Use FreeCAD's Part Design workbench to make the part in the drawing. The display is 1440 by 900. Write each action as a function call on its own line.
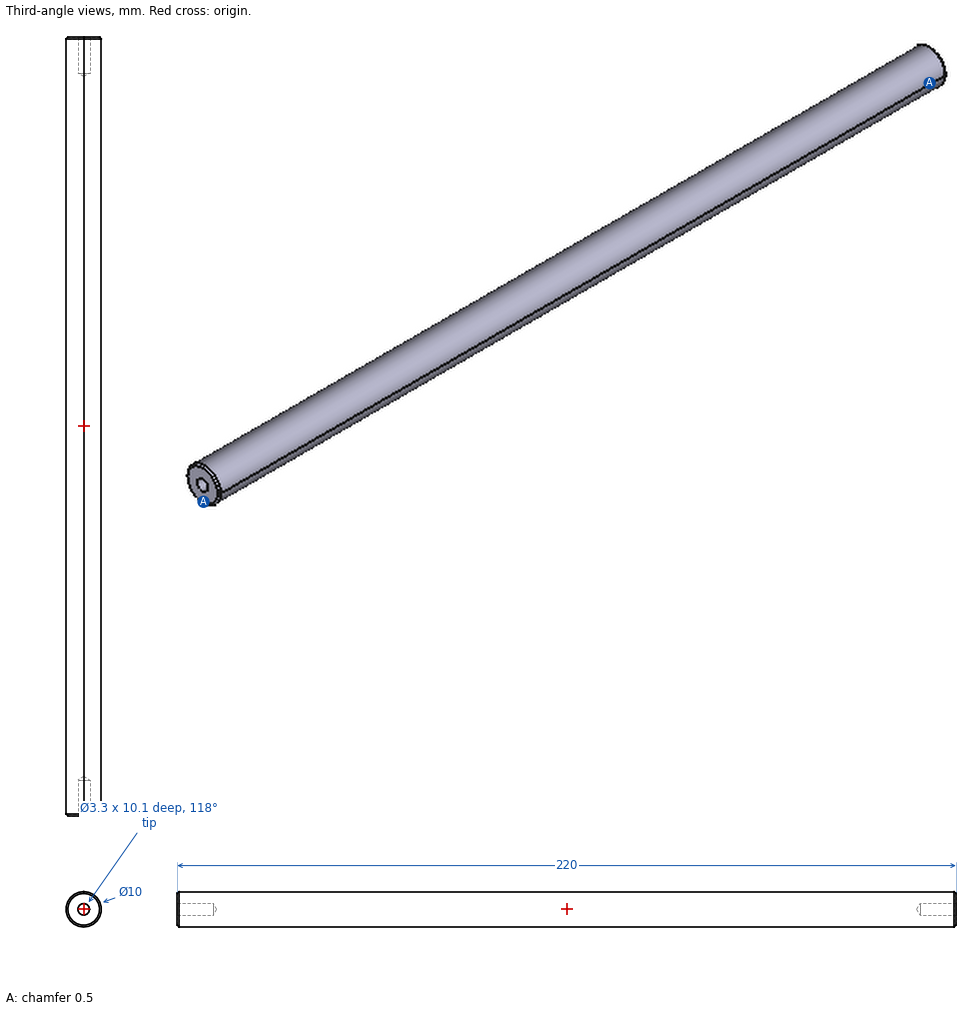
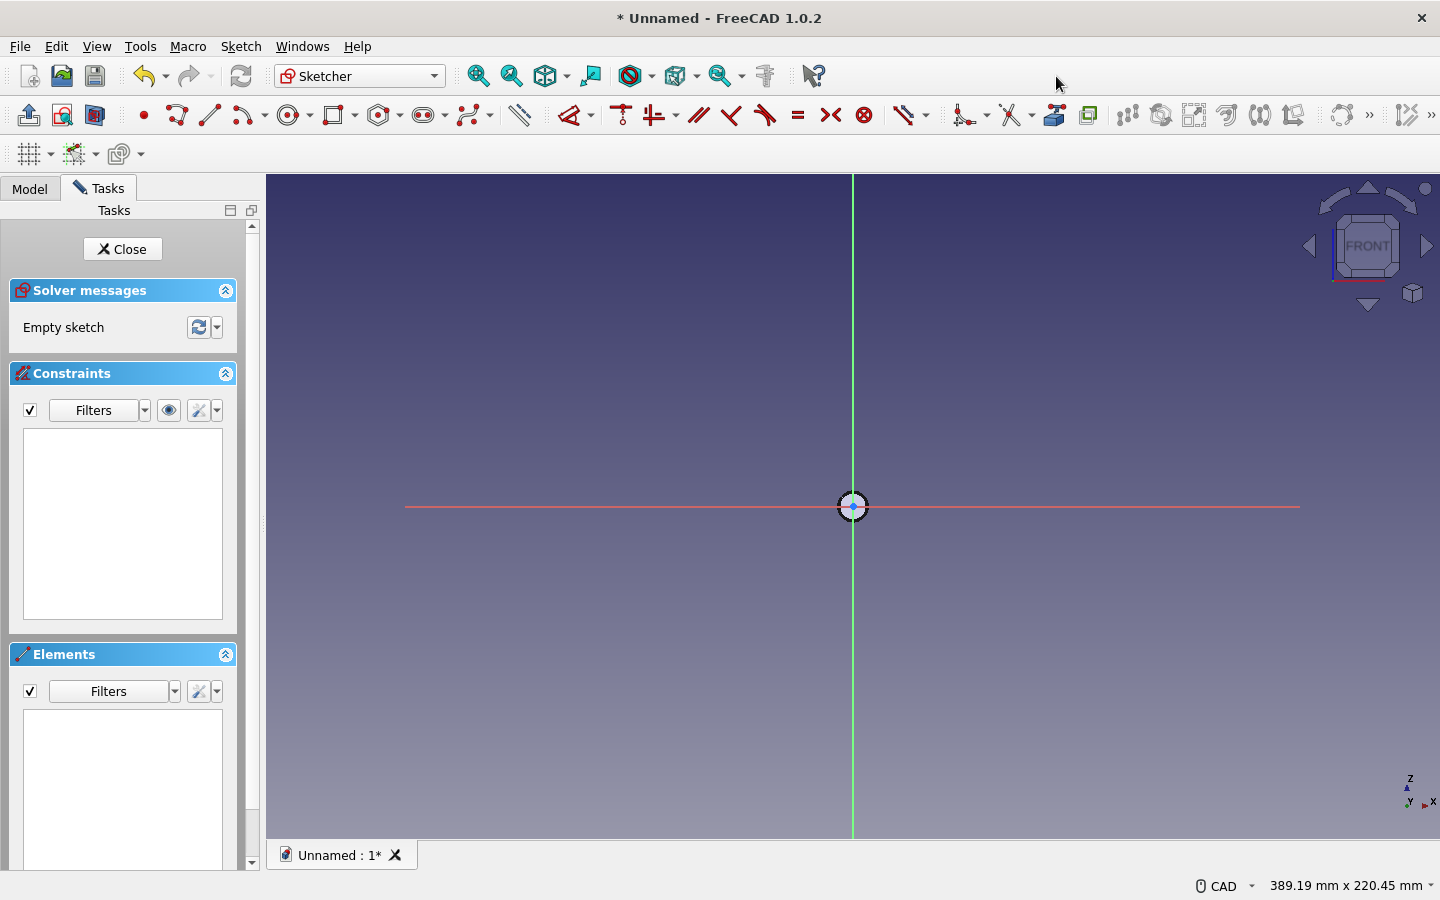
scroll(857, 506, up, 15)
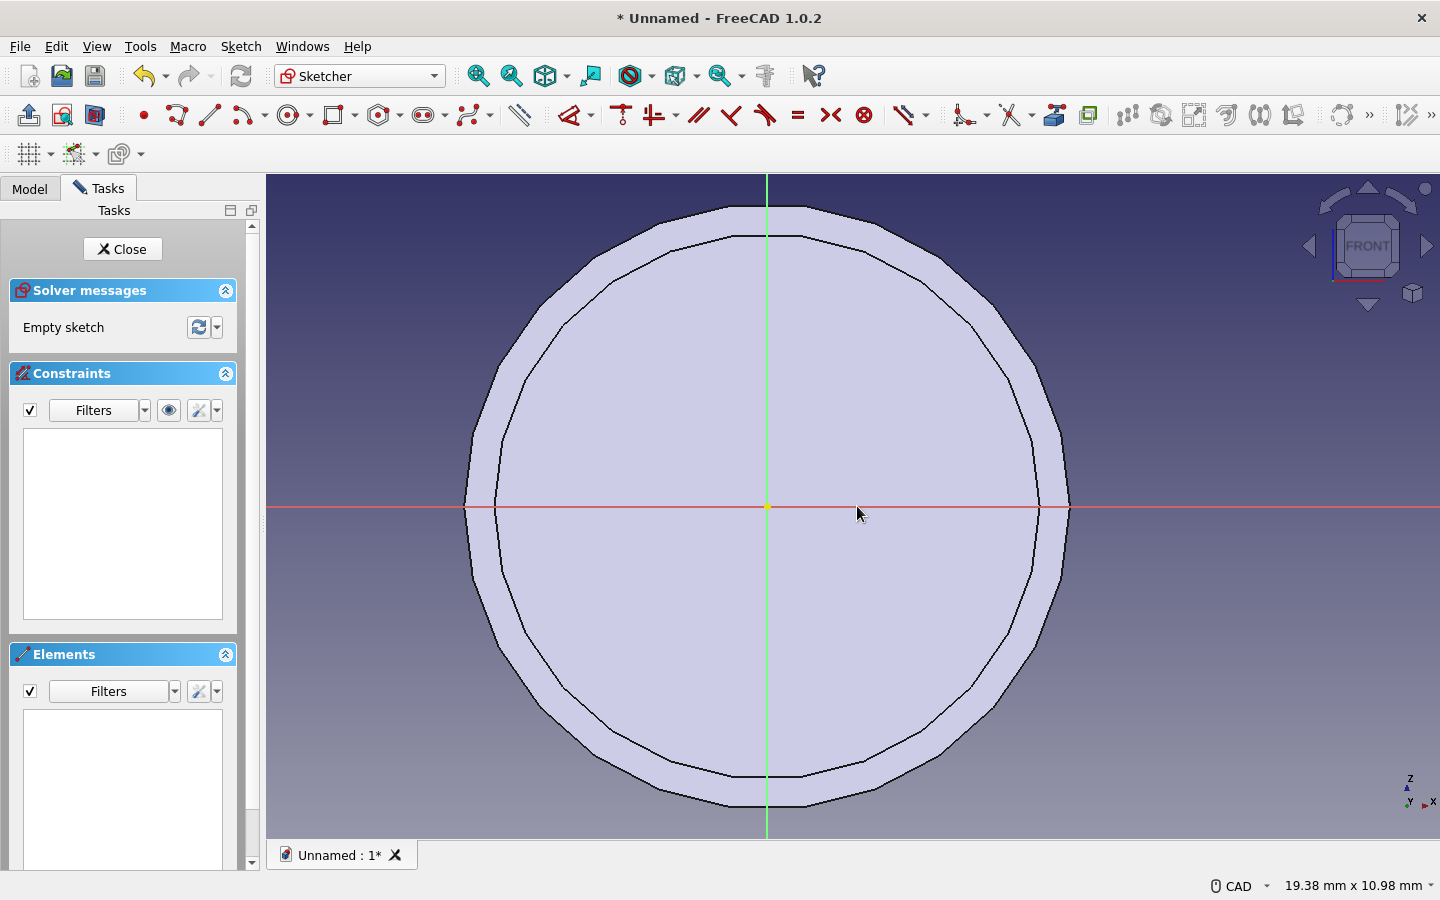
scroll(753, 506, up, 4)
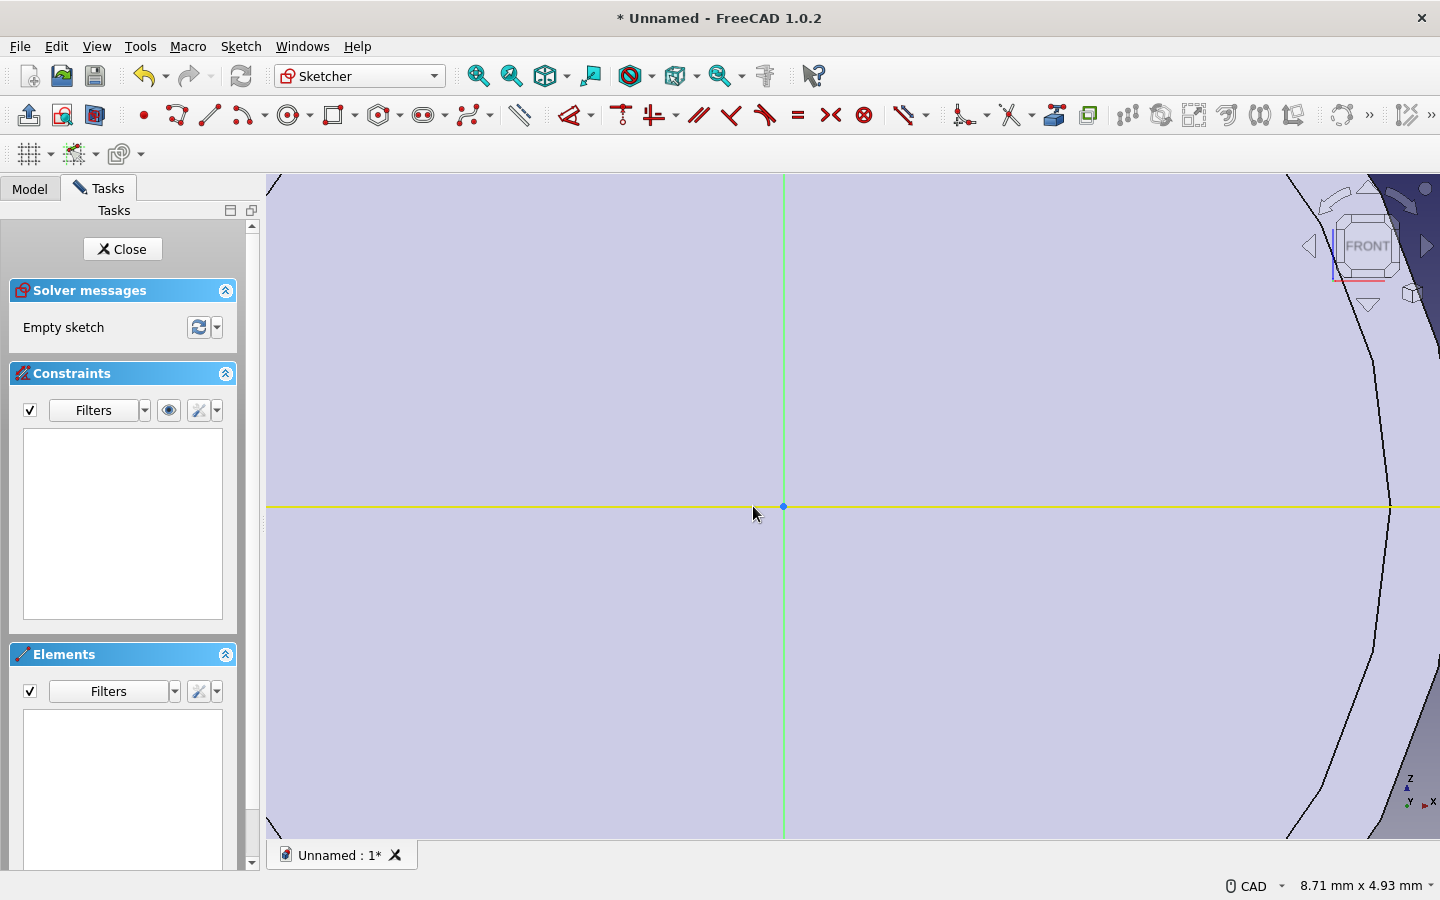
key(g)
key(c)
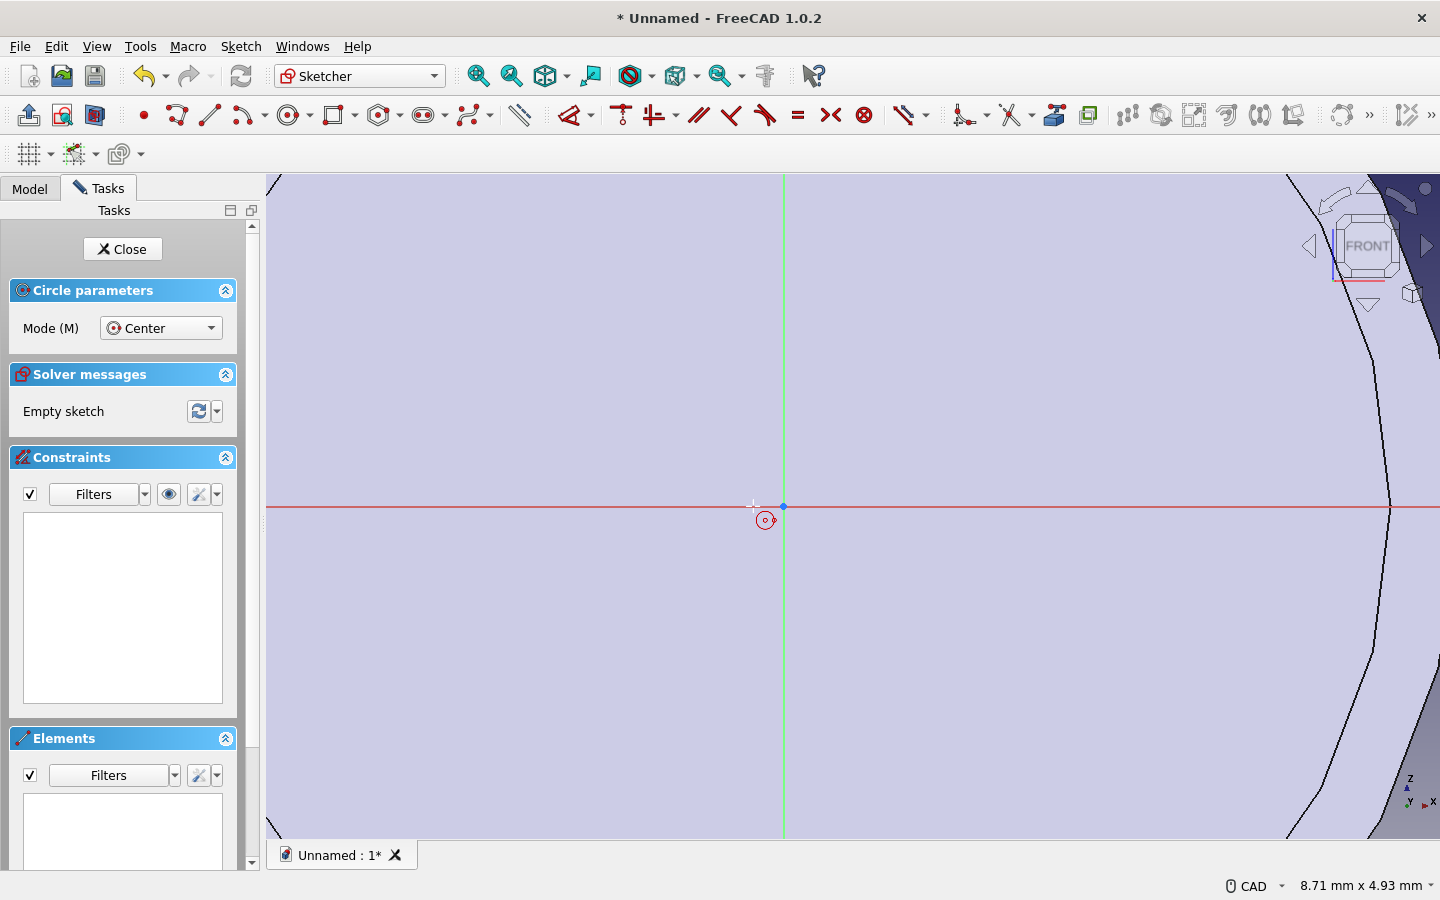
click(784, 506)
move(941, 349)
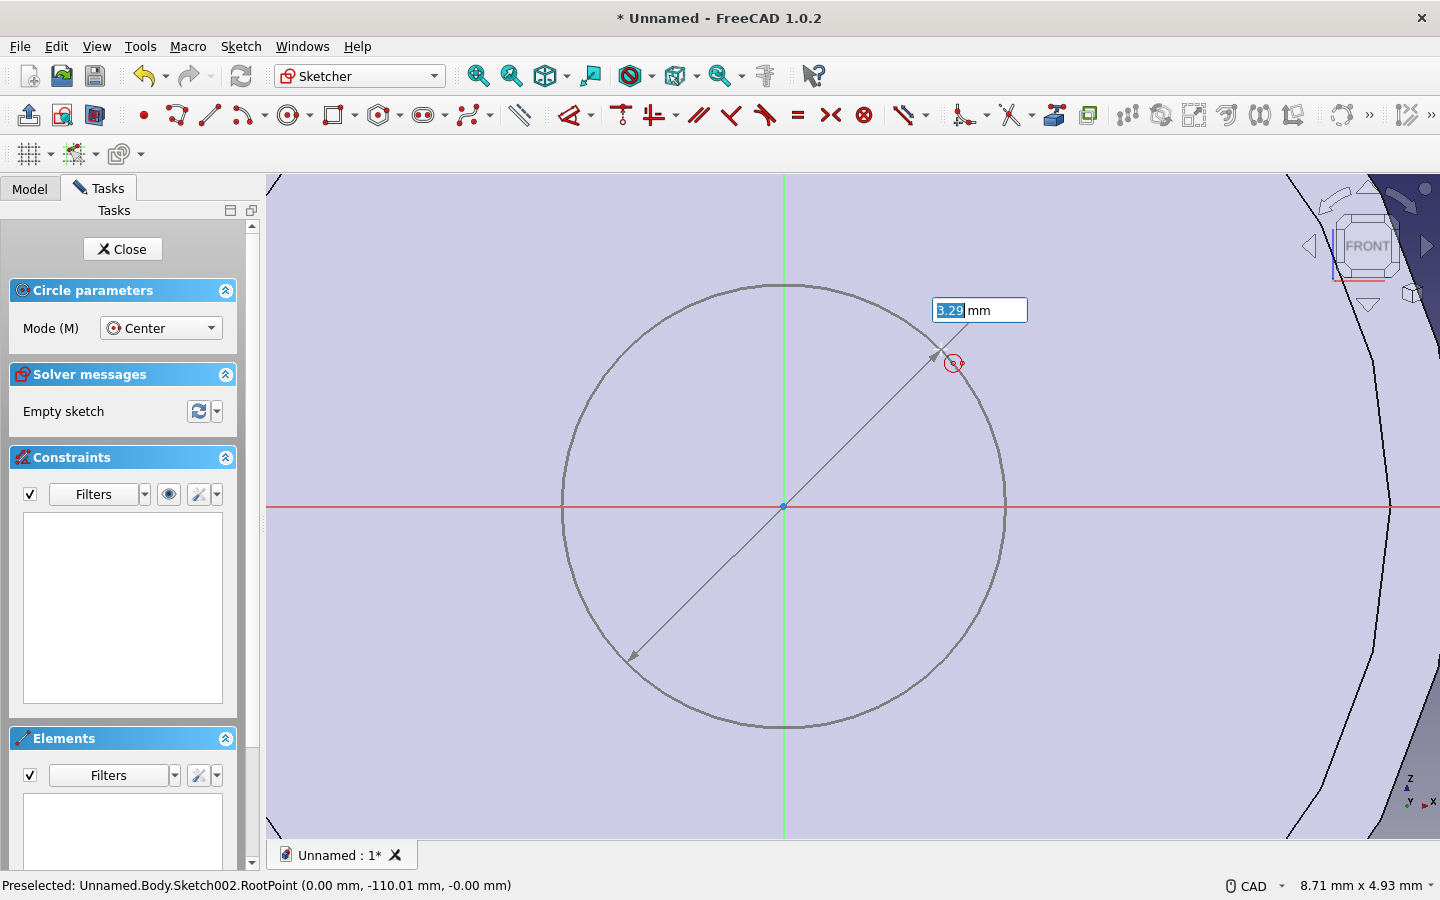
text(3.3)
key(Return)
key(Escape)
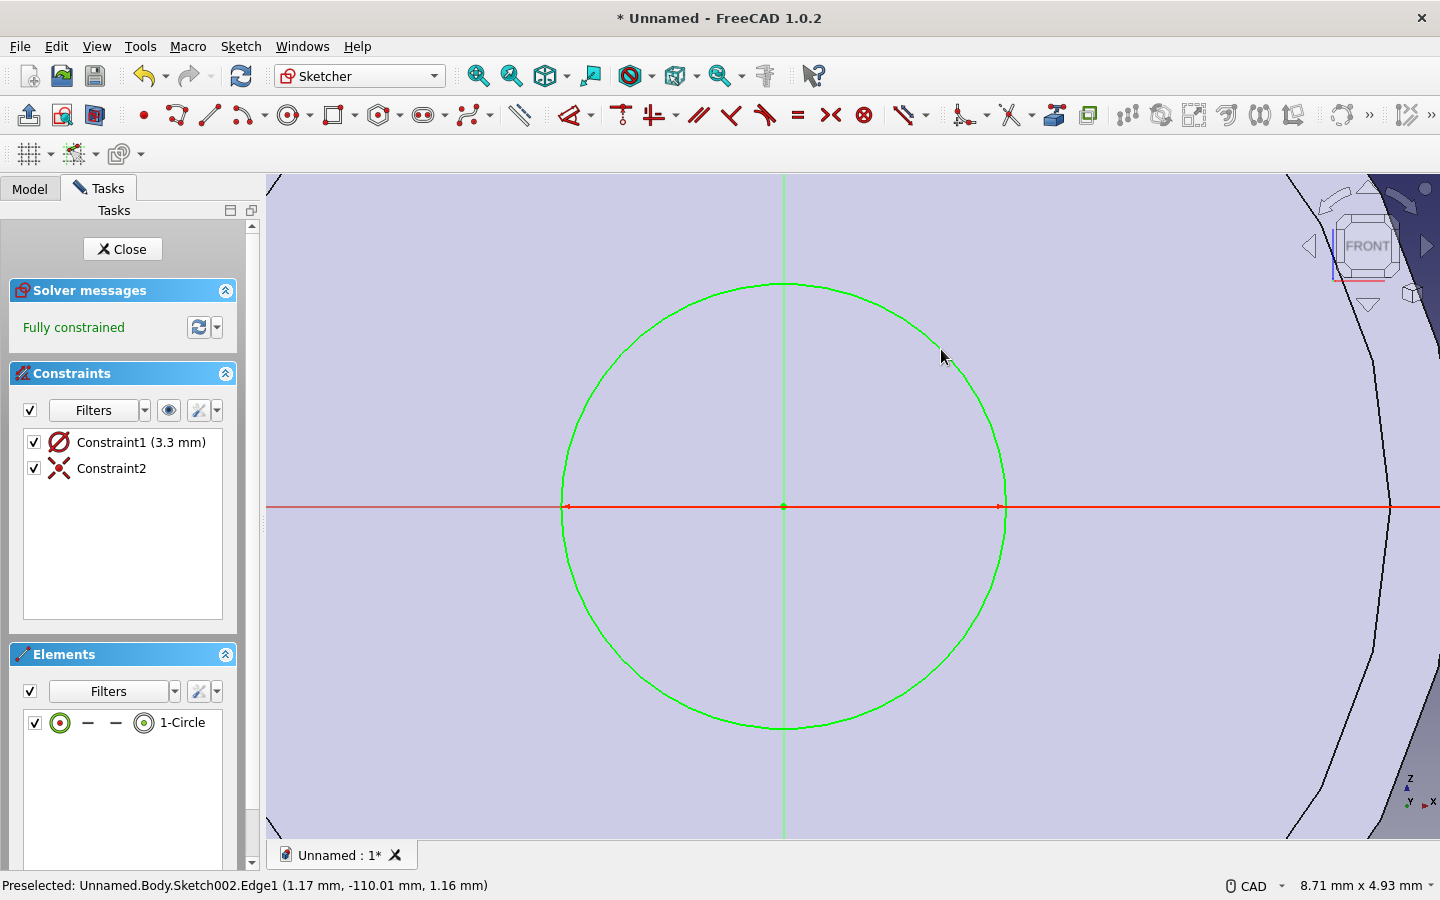
click(123, 249)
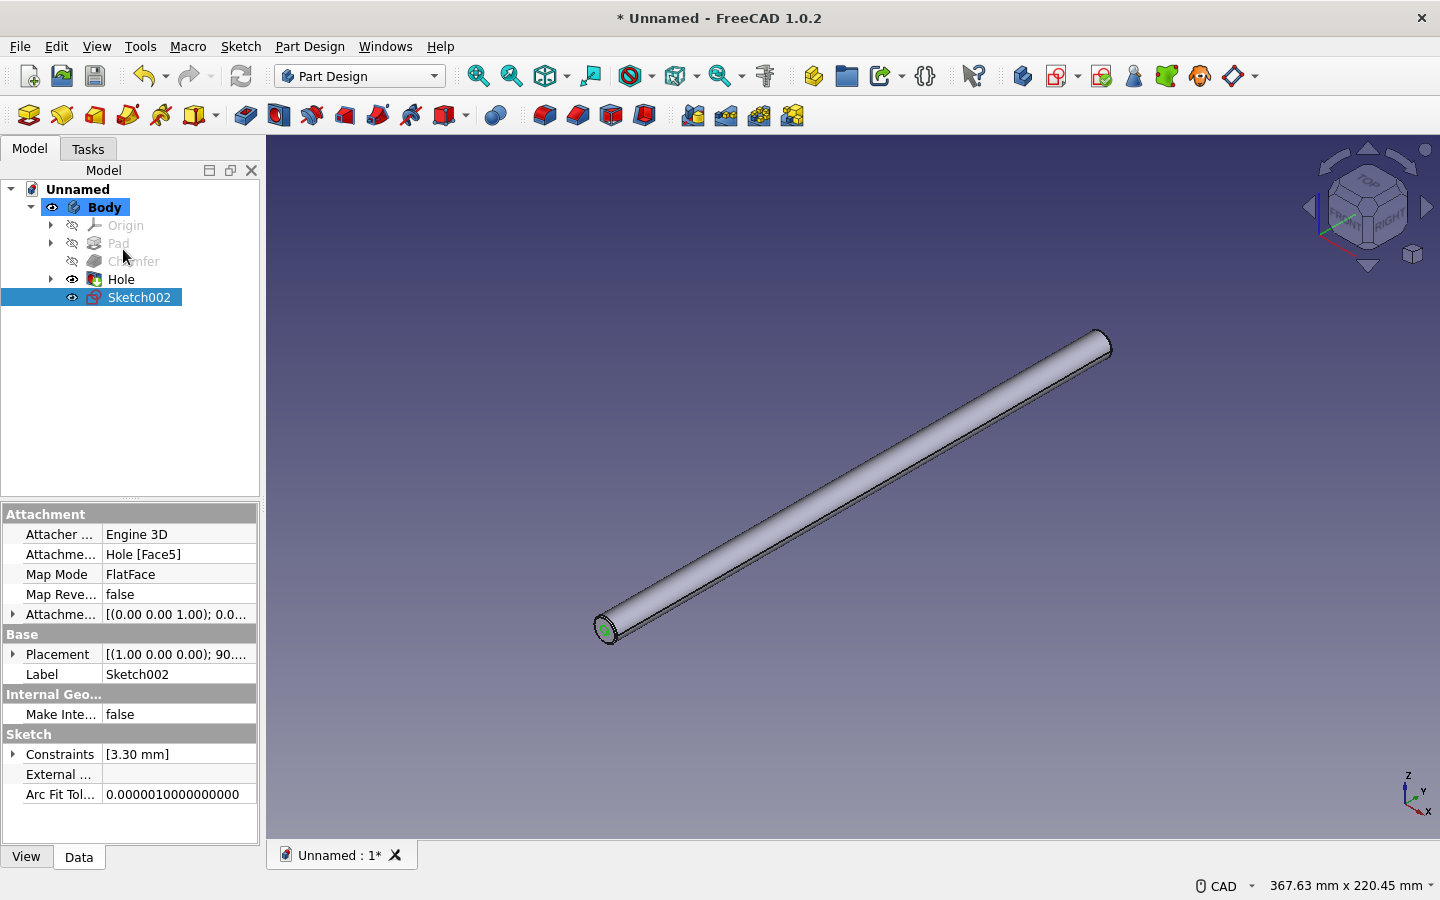
click(279, 116)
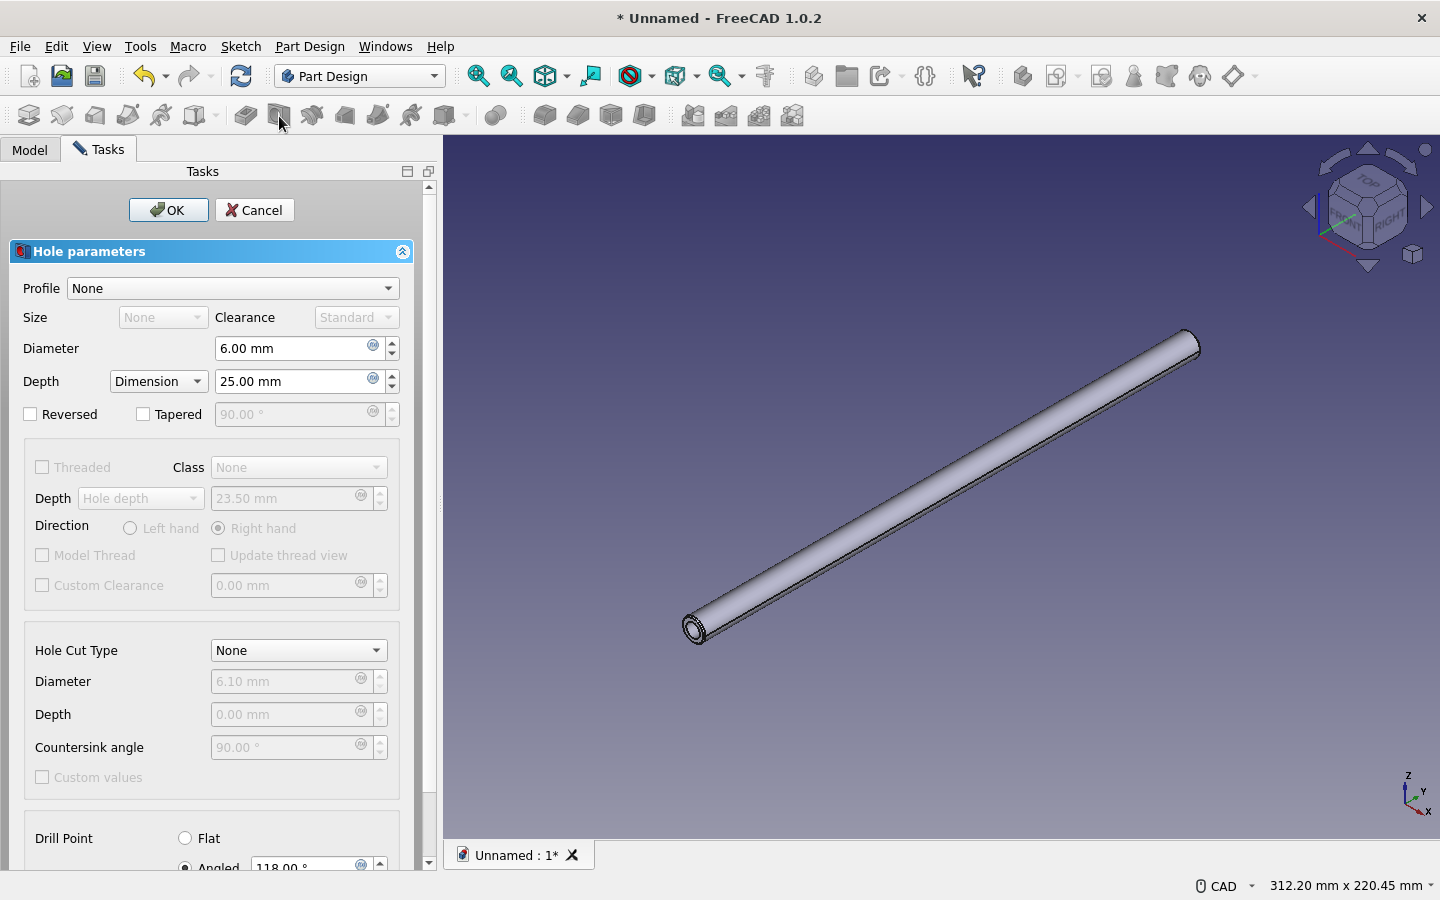
triple_click(300, 348)